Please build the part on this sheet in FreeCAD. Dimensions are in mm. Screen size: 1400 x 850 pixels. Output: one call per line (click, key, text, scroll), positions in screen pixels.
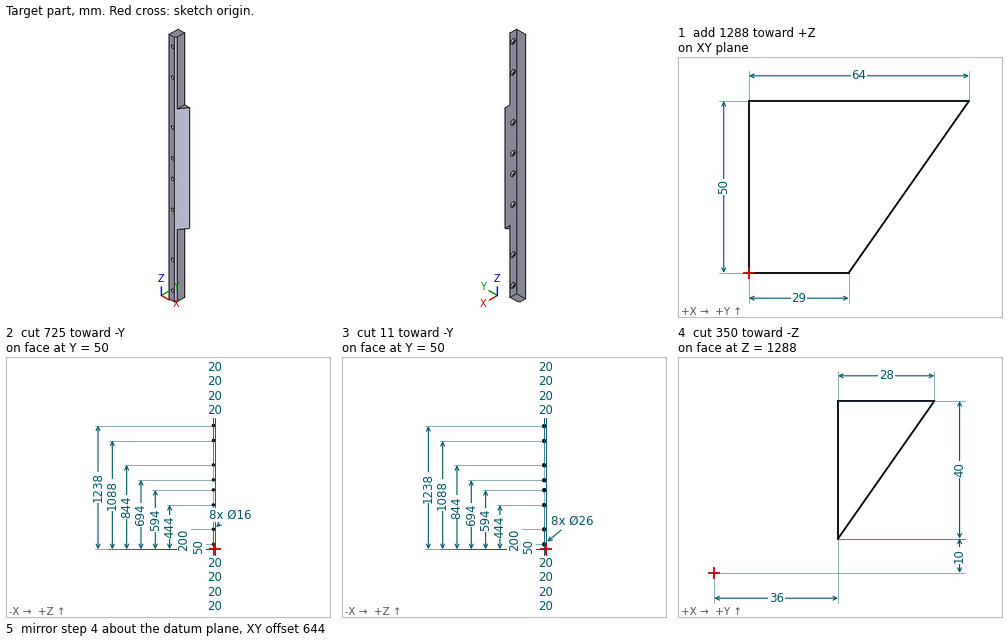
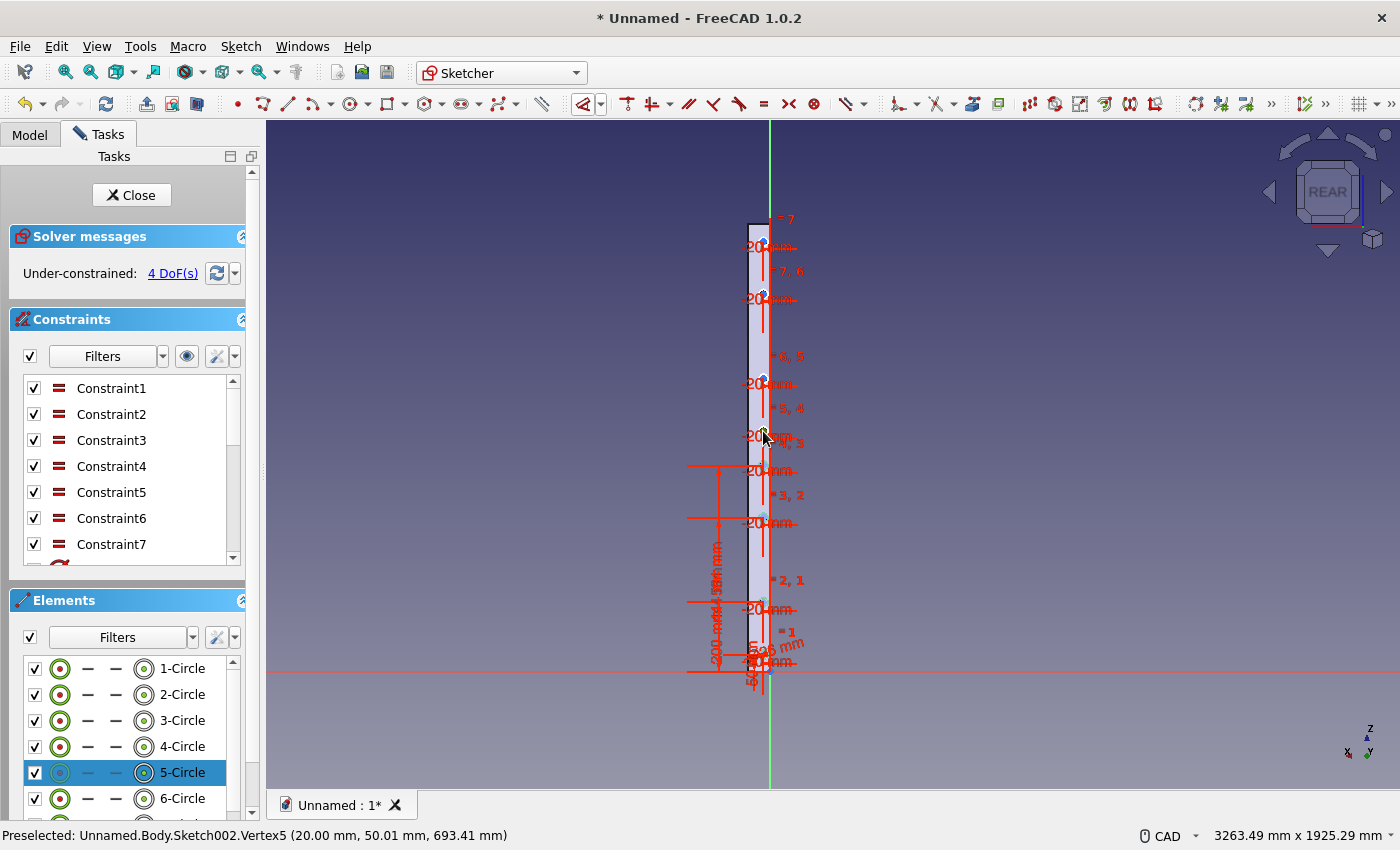
key(i)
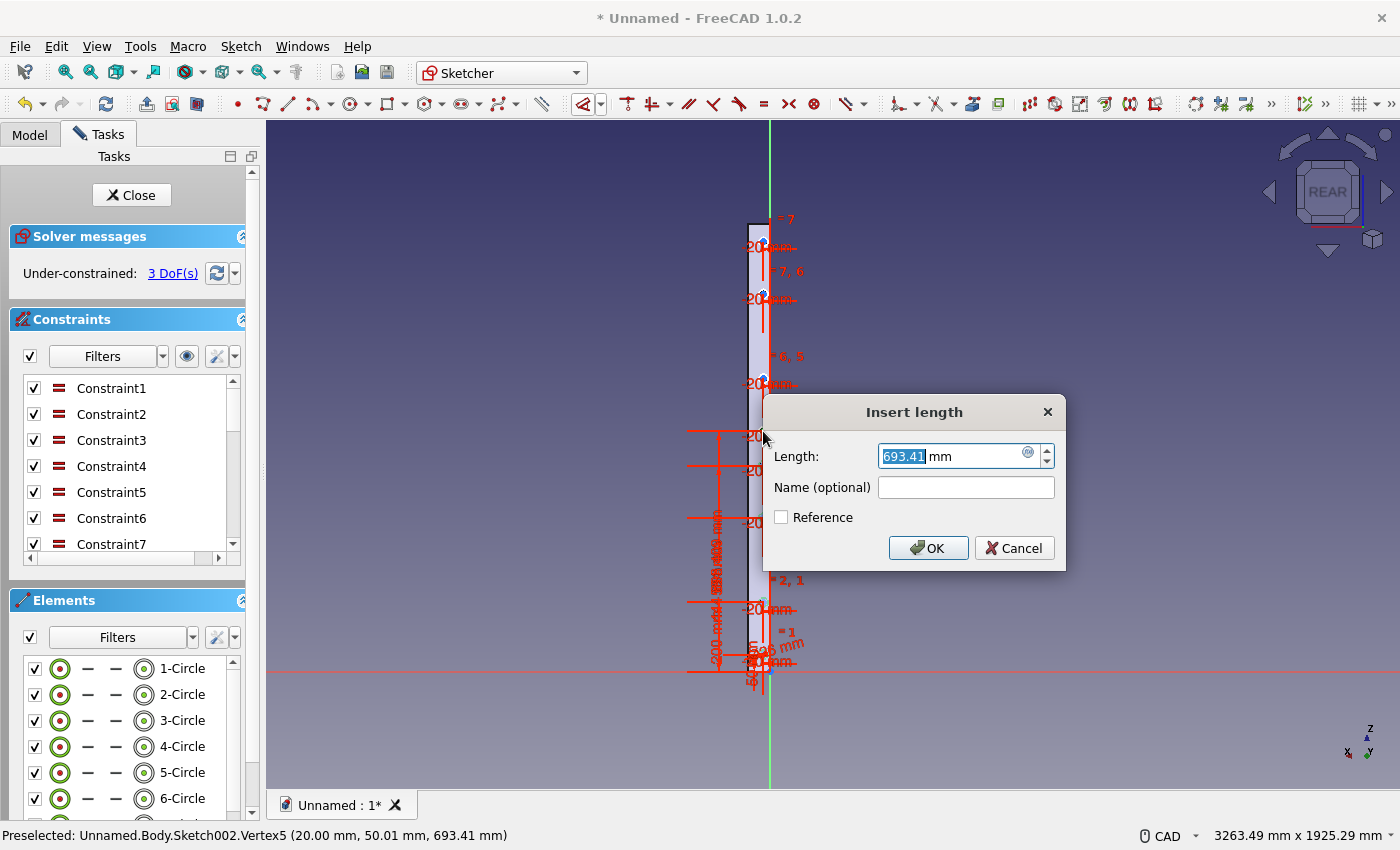
text(694)
key(Return)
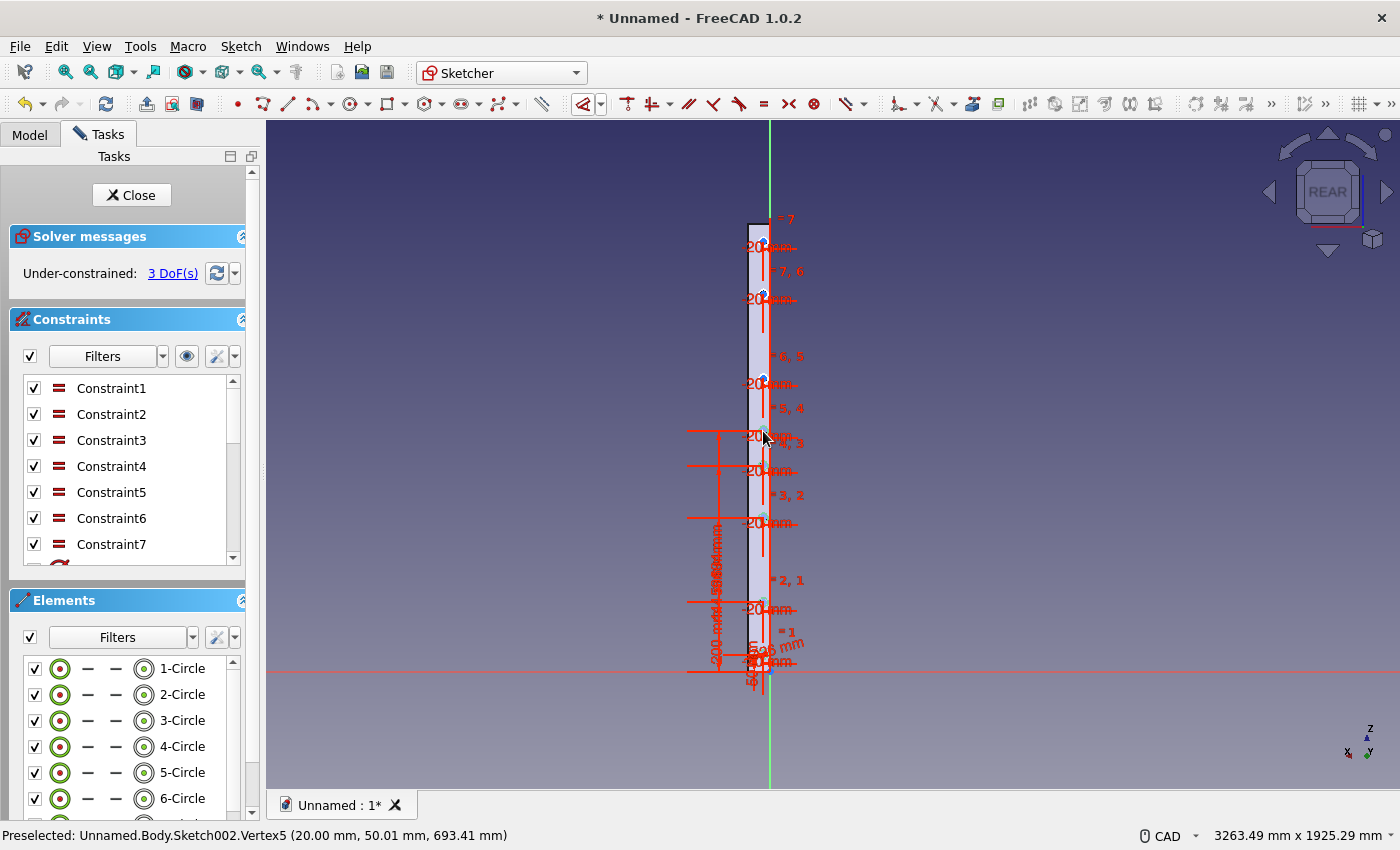
click(763, 379)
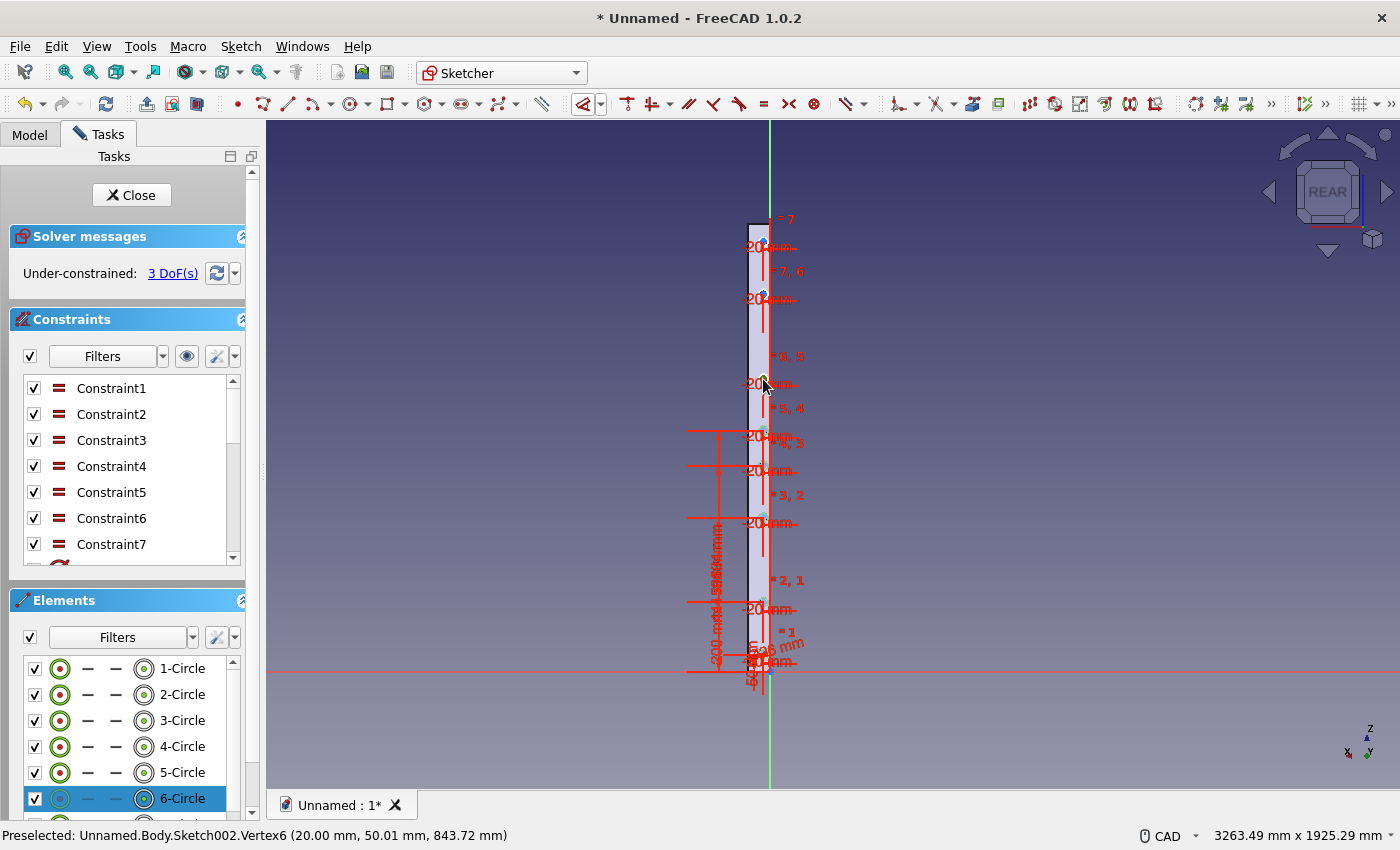
key(i)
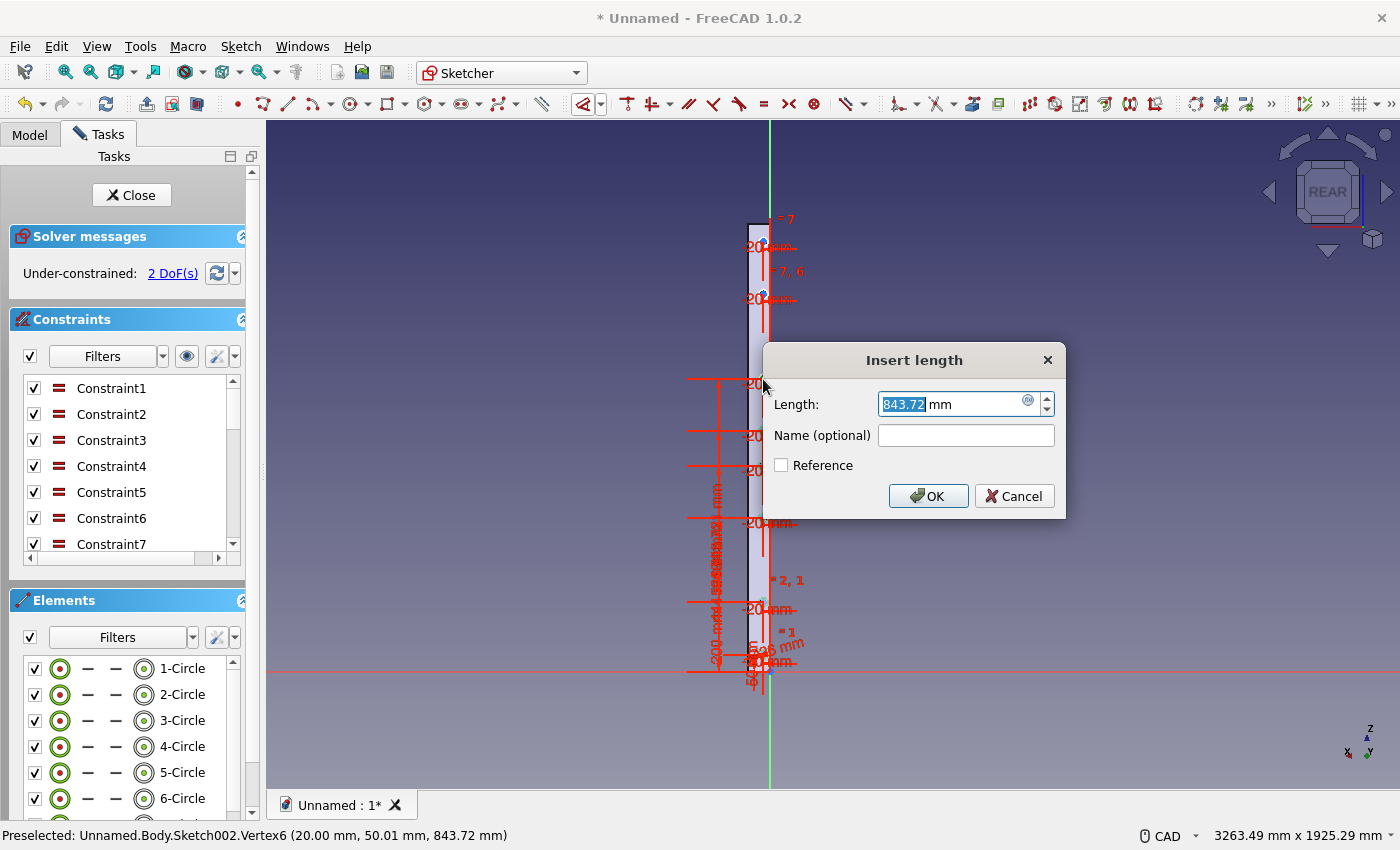
text(844)
key(Return)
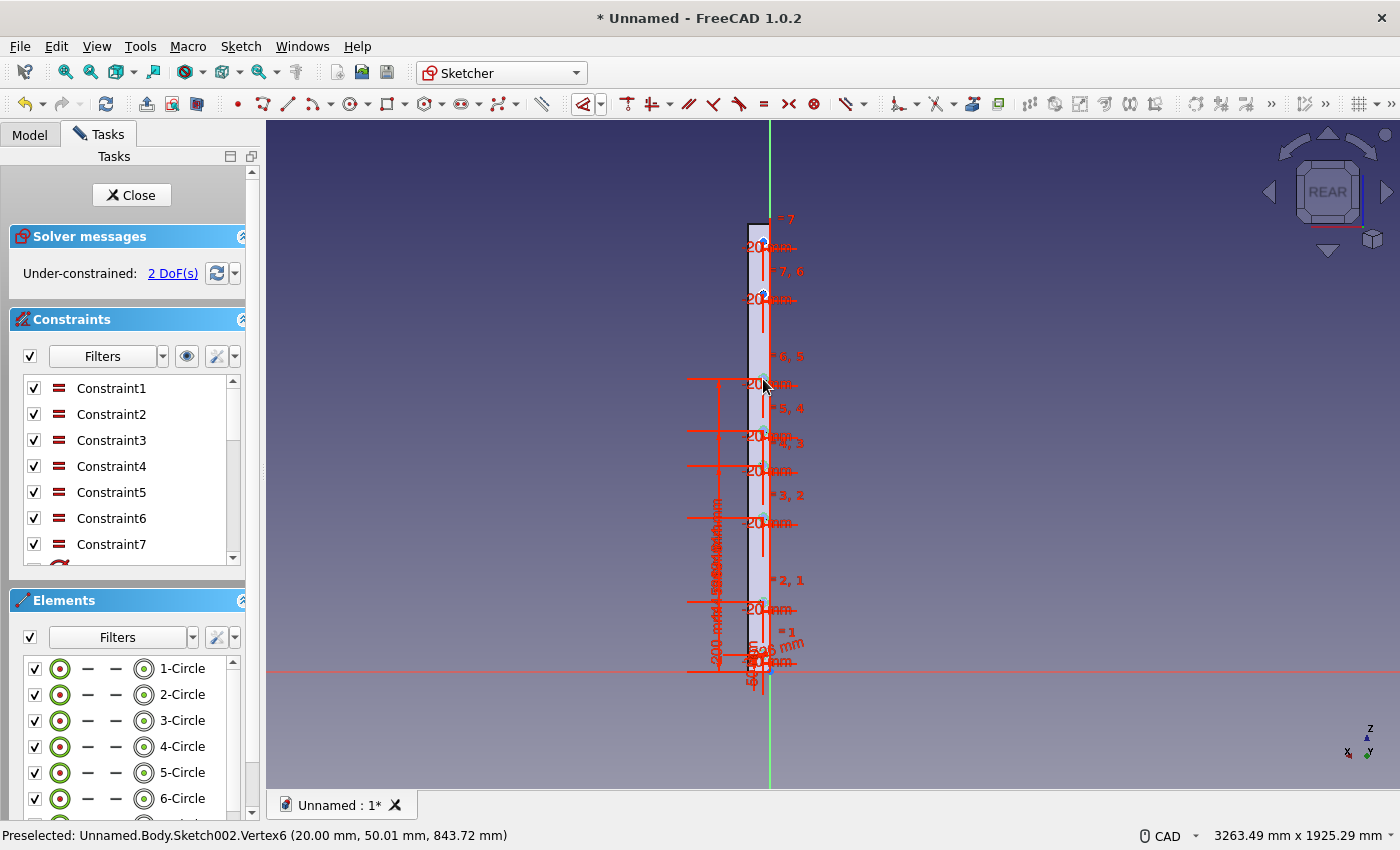
click(763, 294)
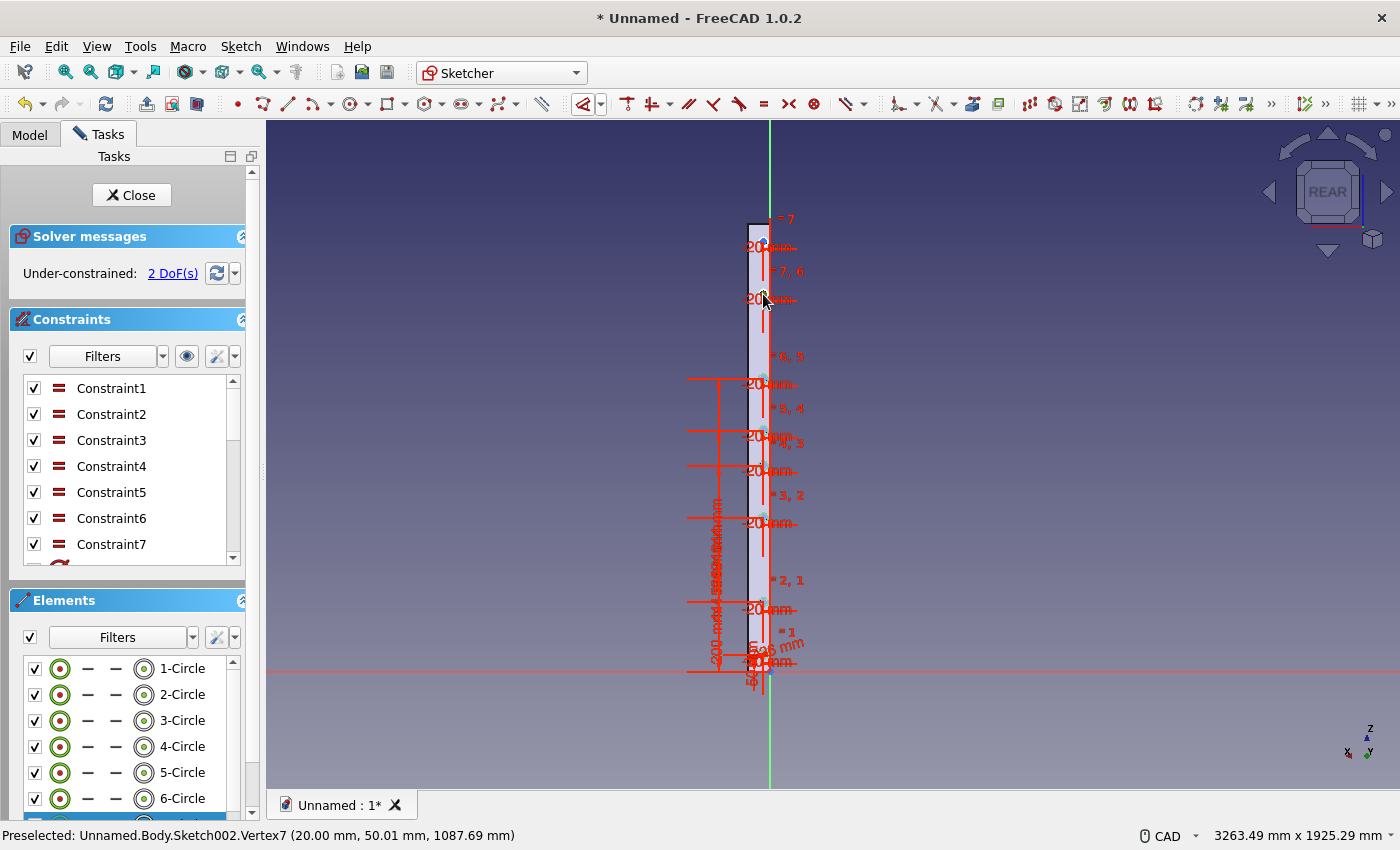
key(i)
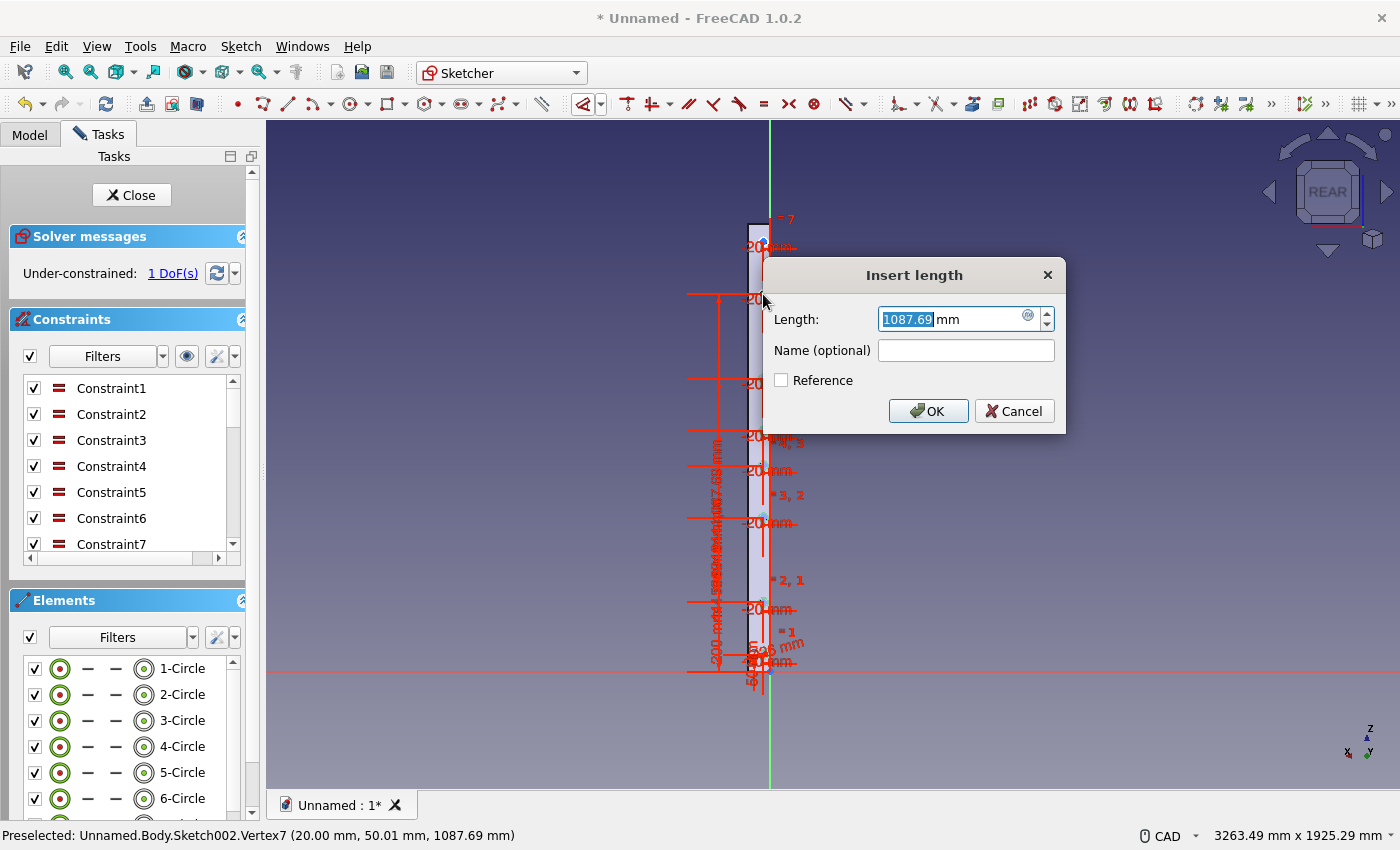
text(1088)
key(Return)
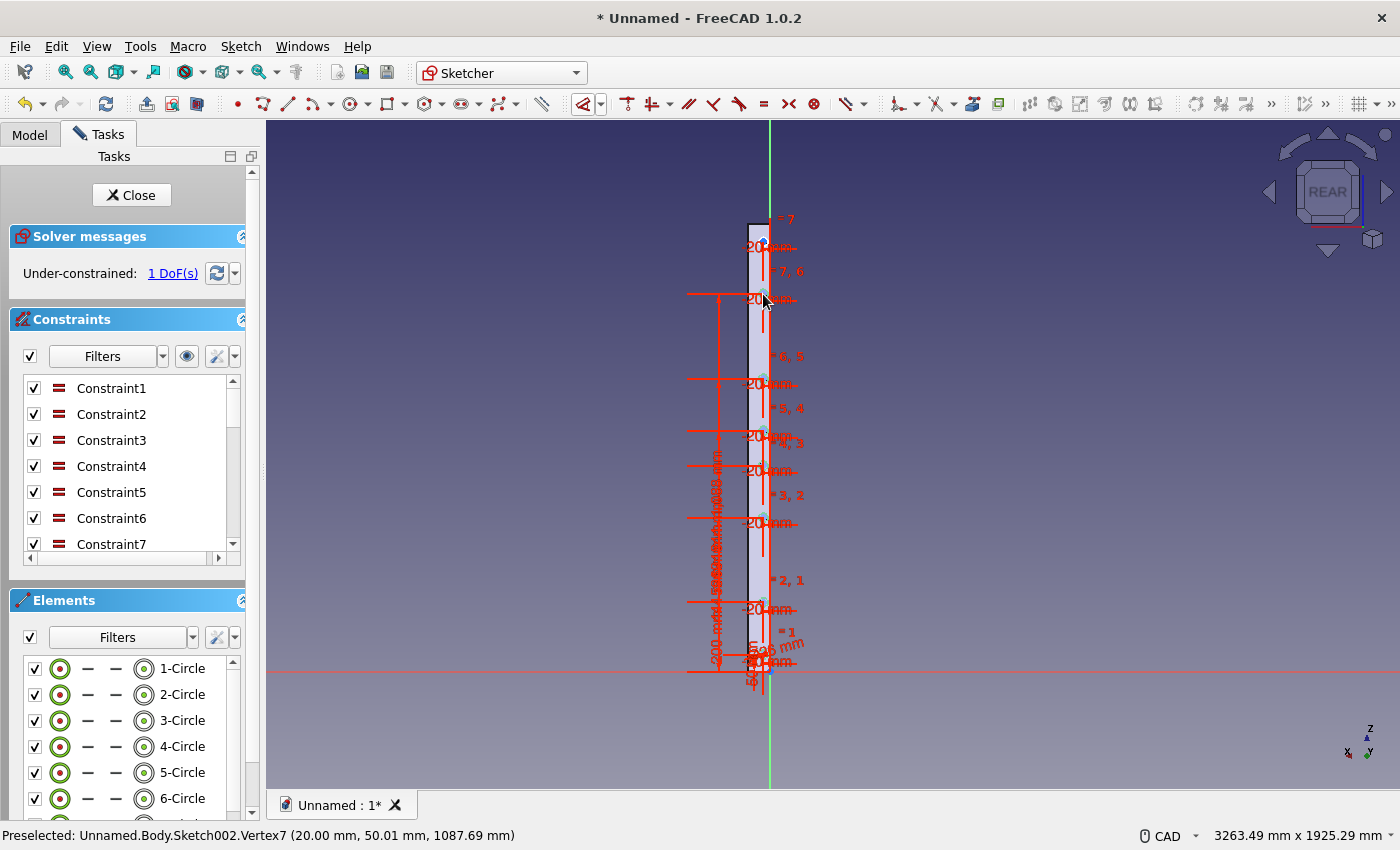
click(763, 242)